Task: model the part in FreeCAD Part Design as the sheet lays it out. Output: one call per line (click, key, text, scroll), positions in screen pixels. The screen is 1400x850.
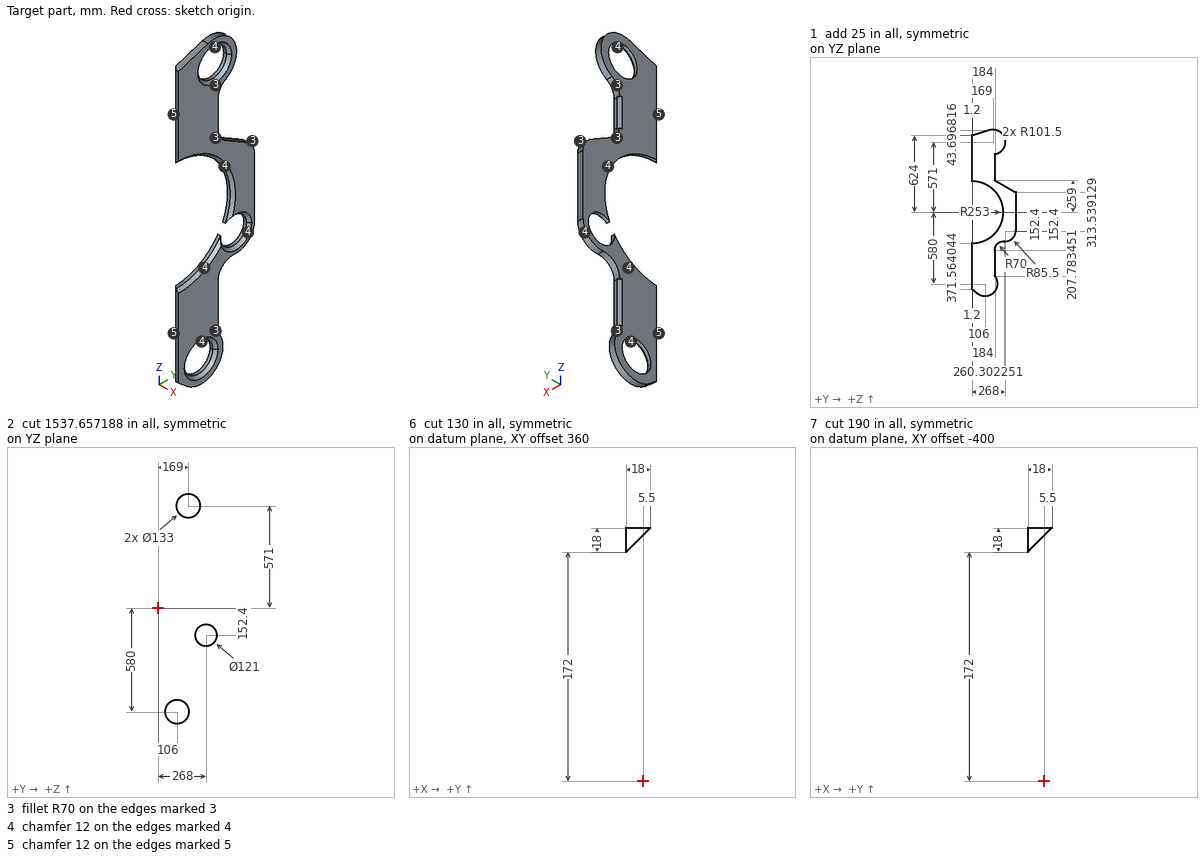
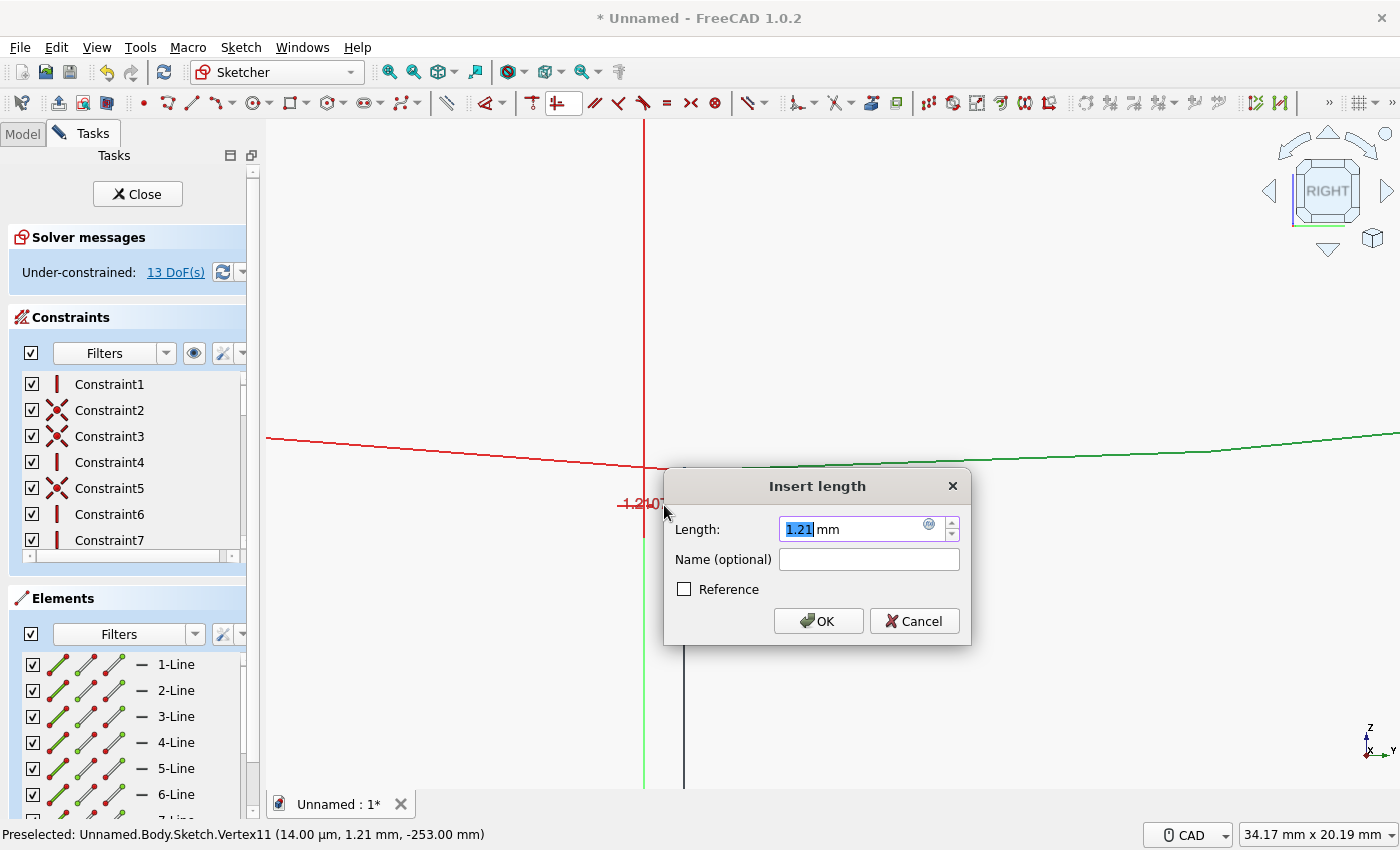
text(1.2)
key(Return)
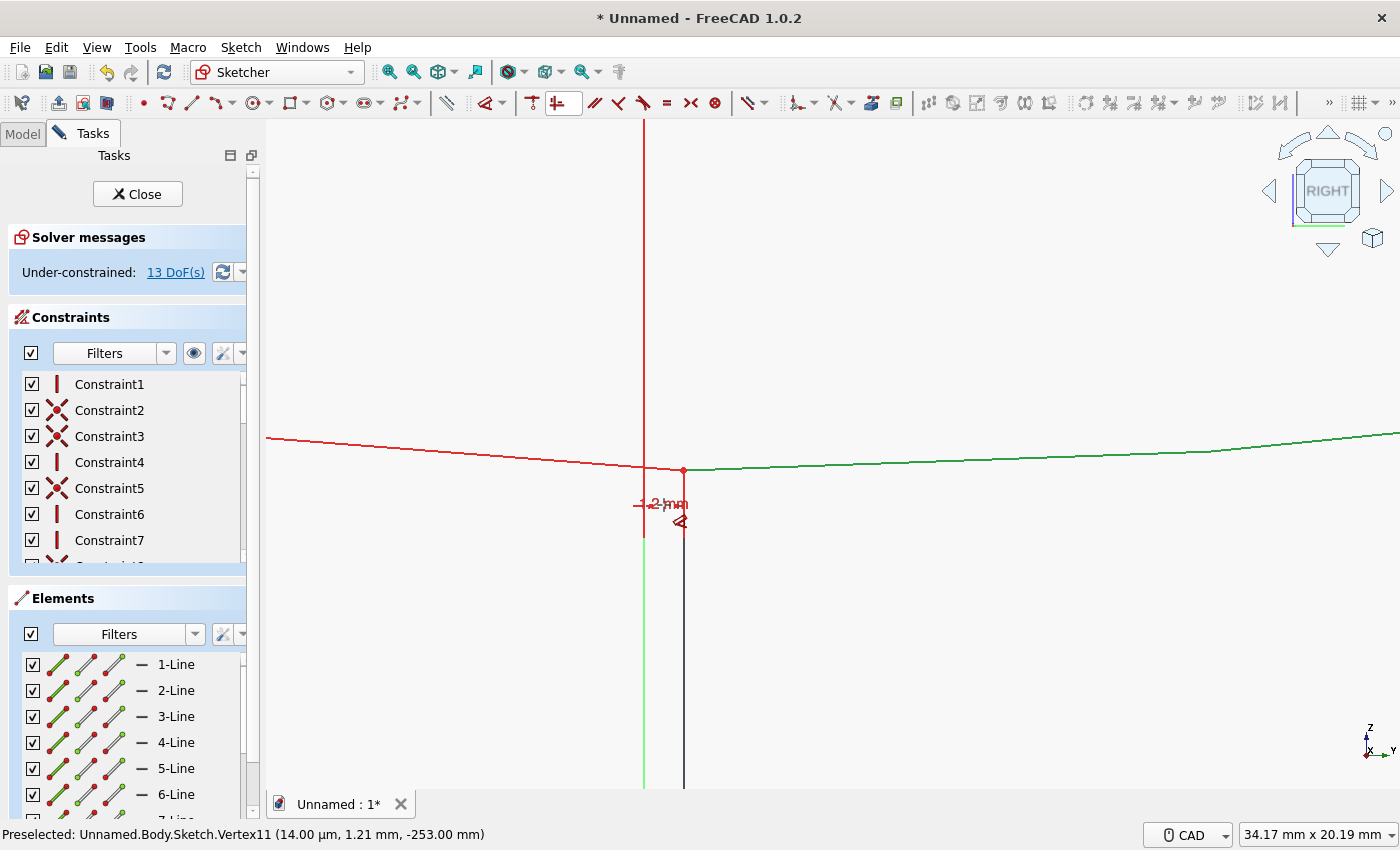
scroll(764, 454, down, 15)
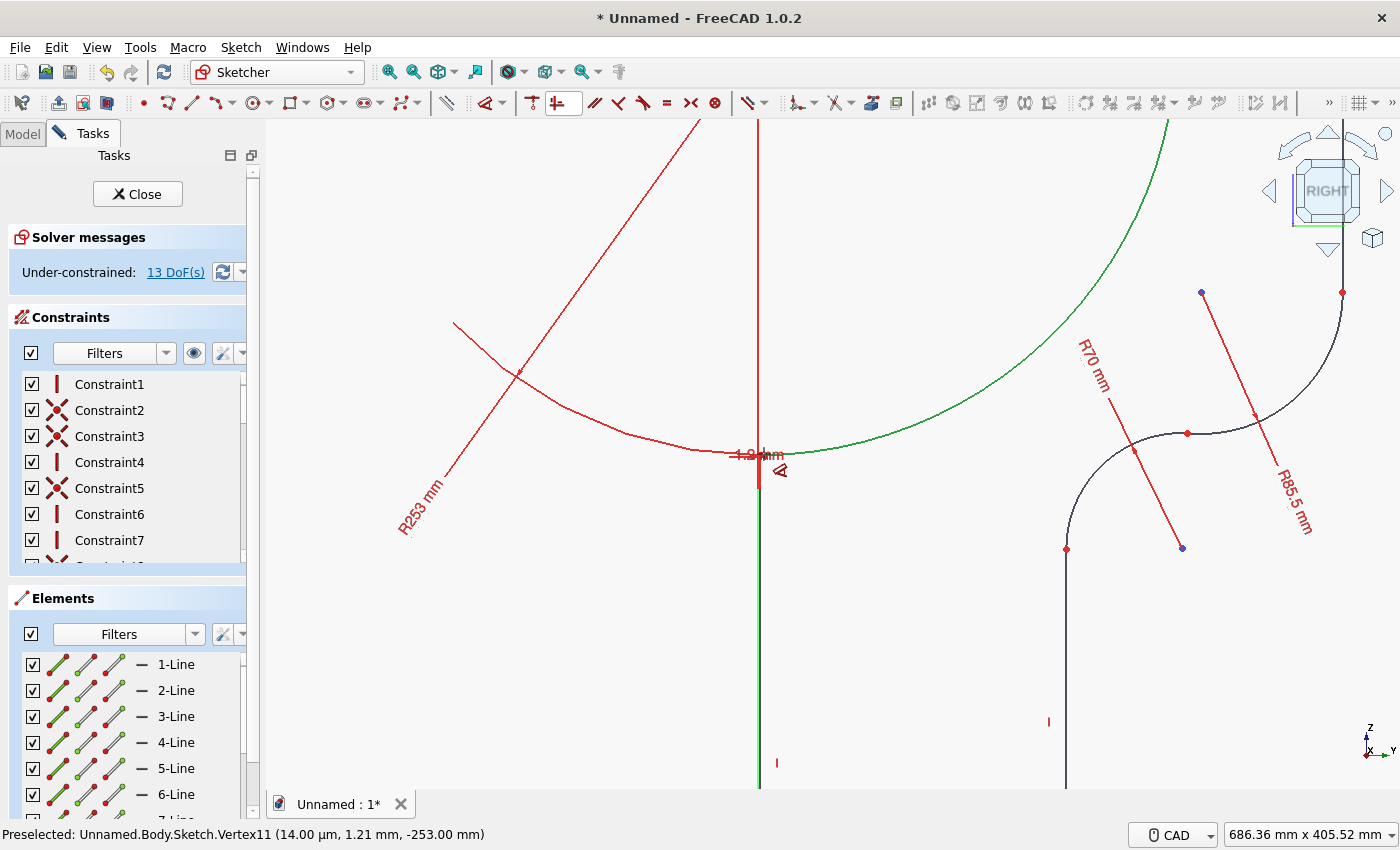
scroll(692, 561, down, 8)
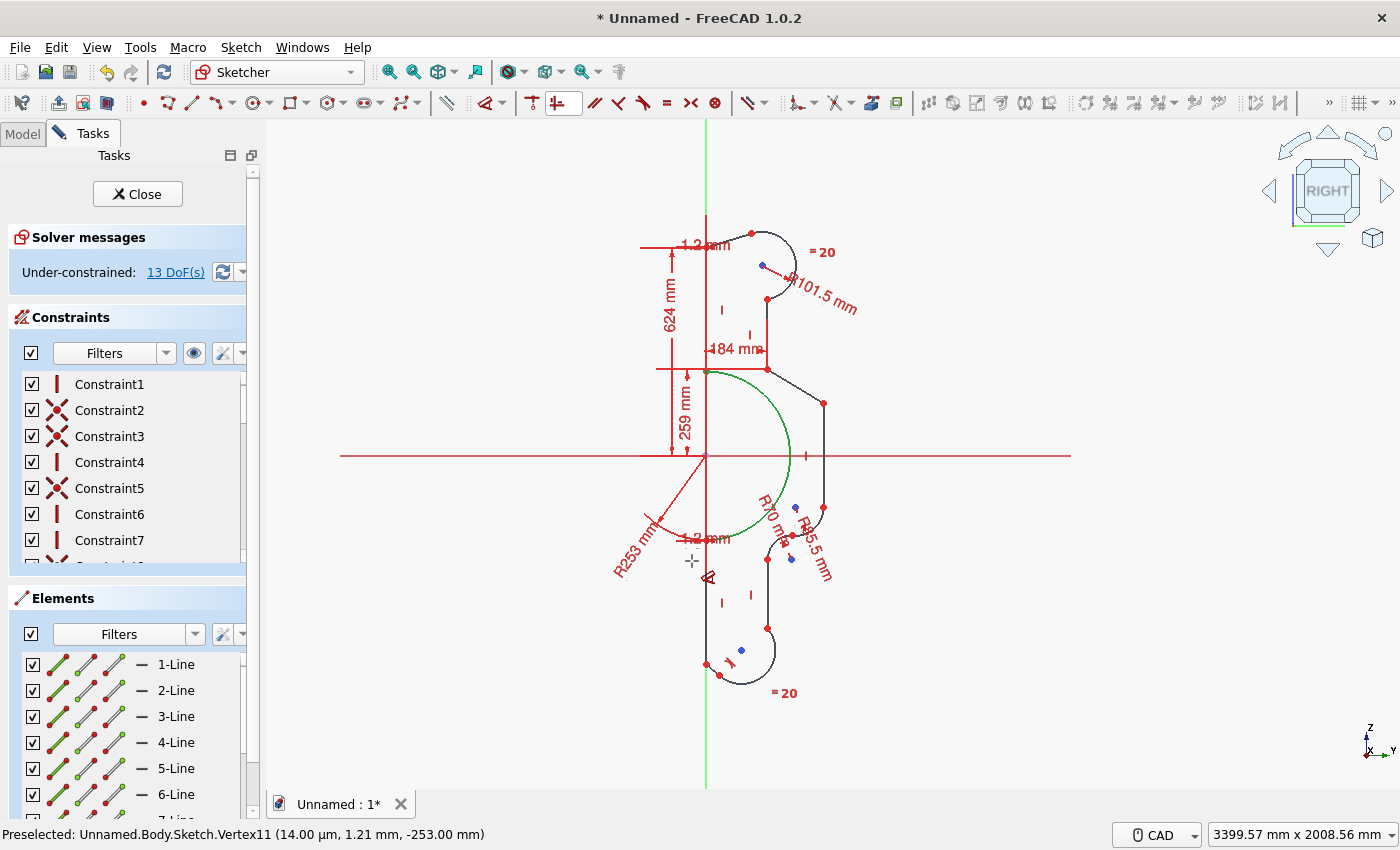
click(768, 629)
click(737, 663)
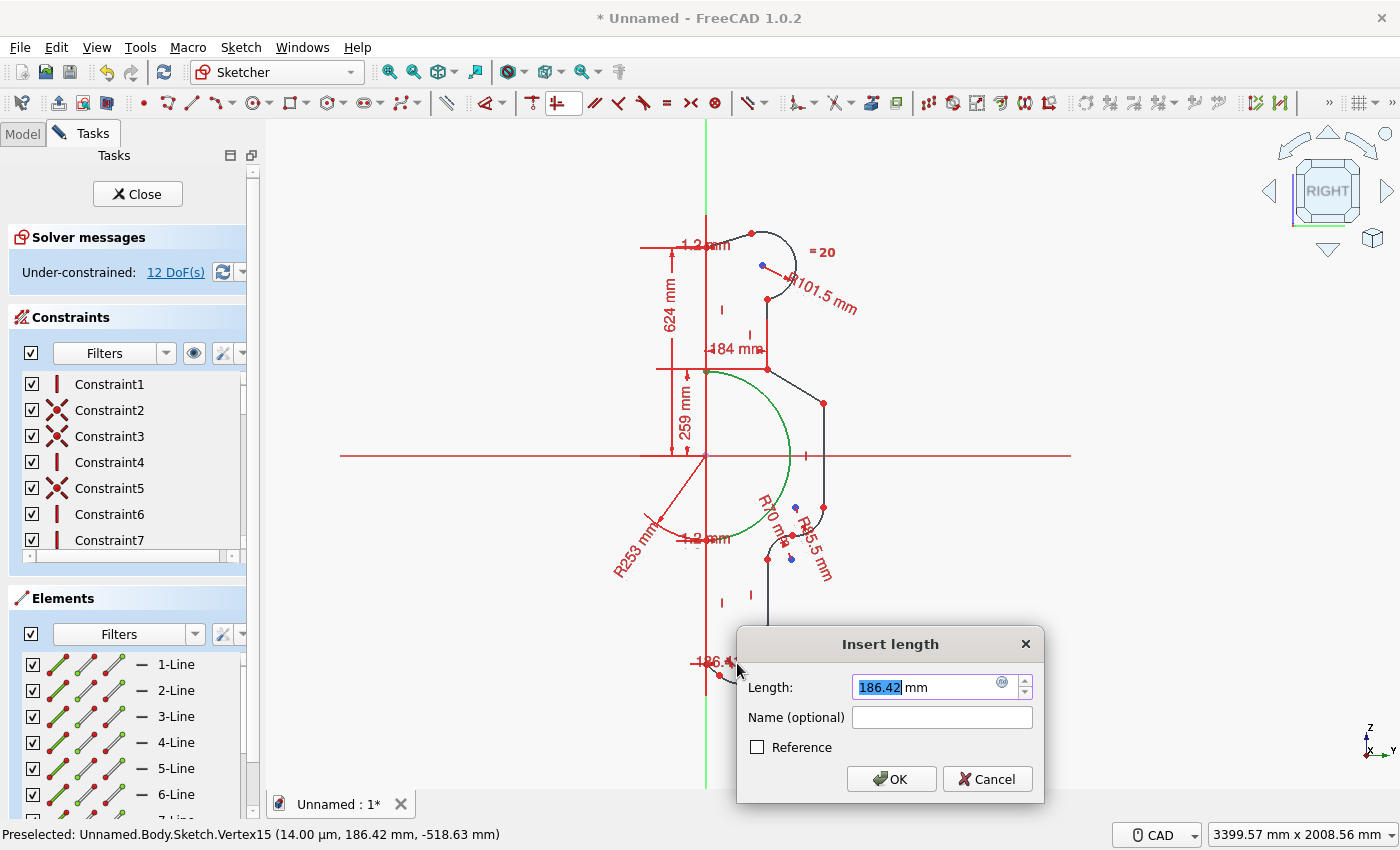
text(184)
key(Return)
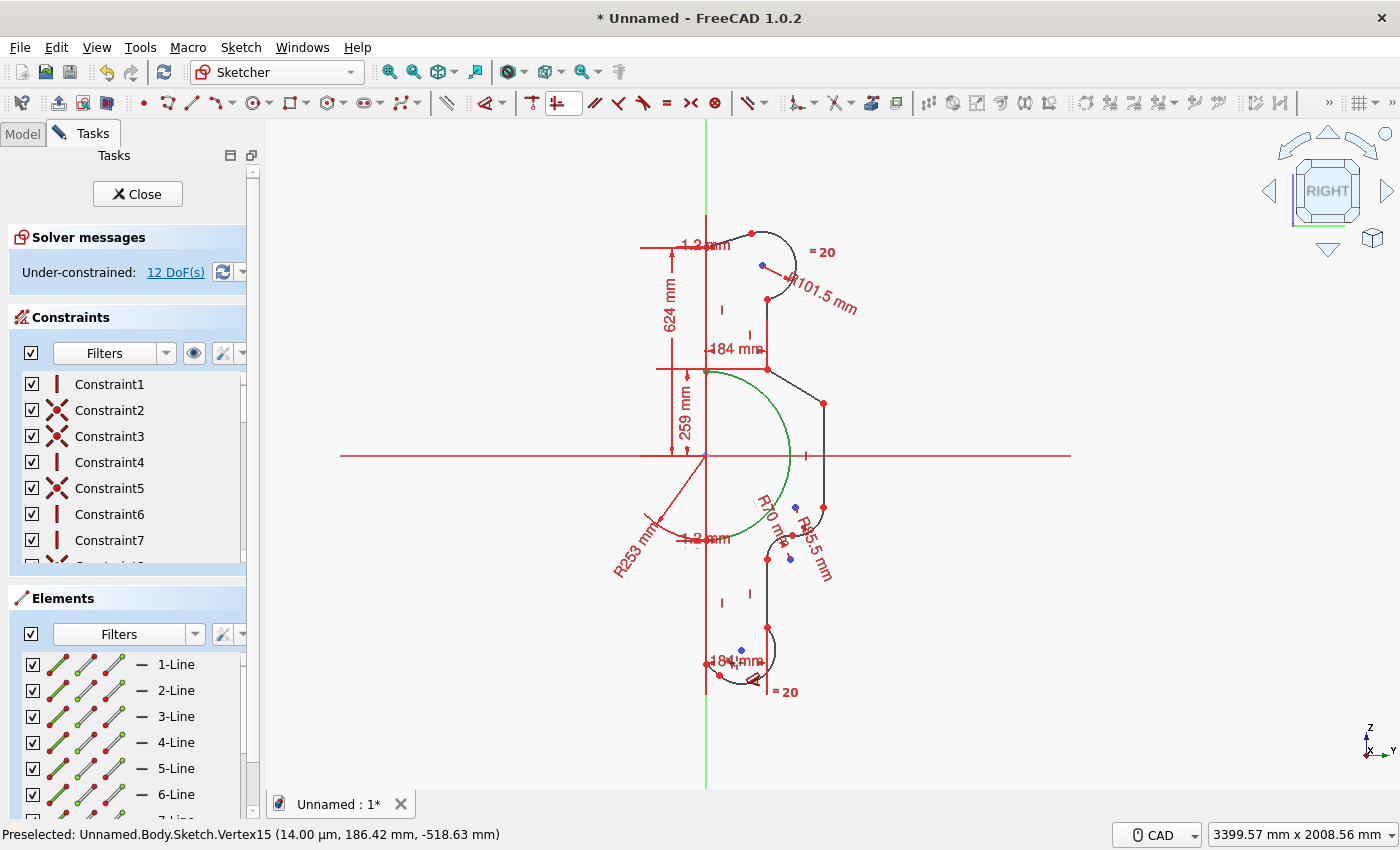
click(762, 266)
click(734, 490)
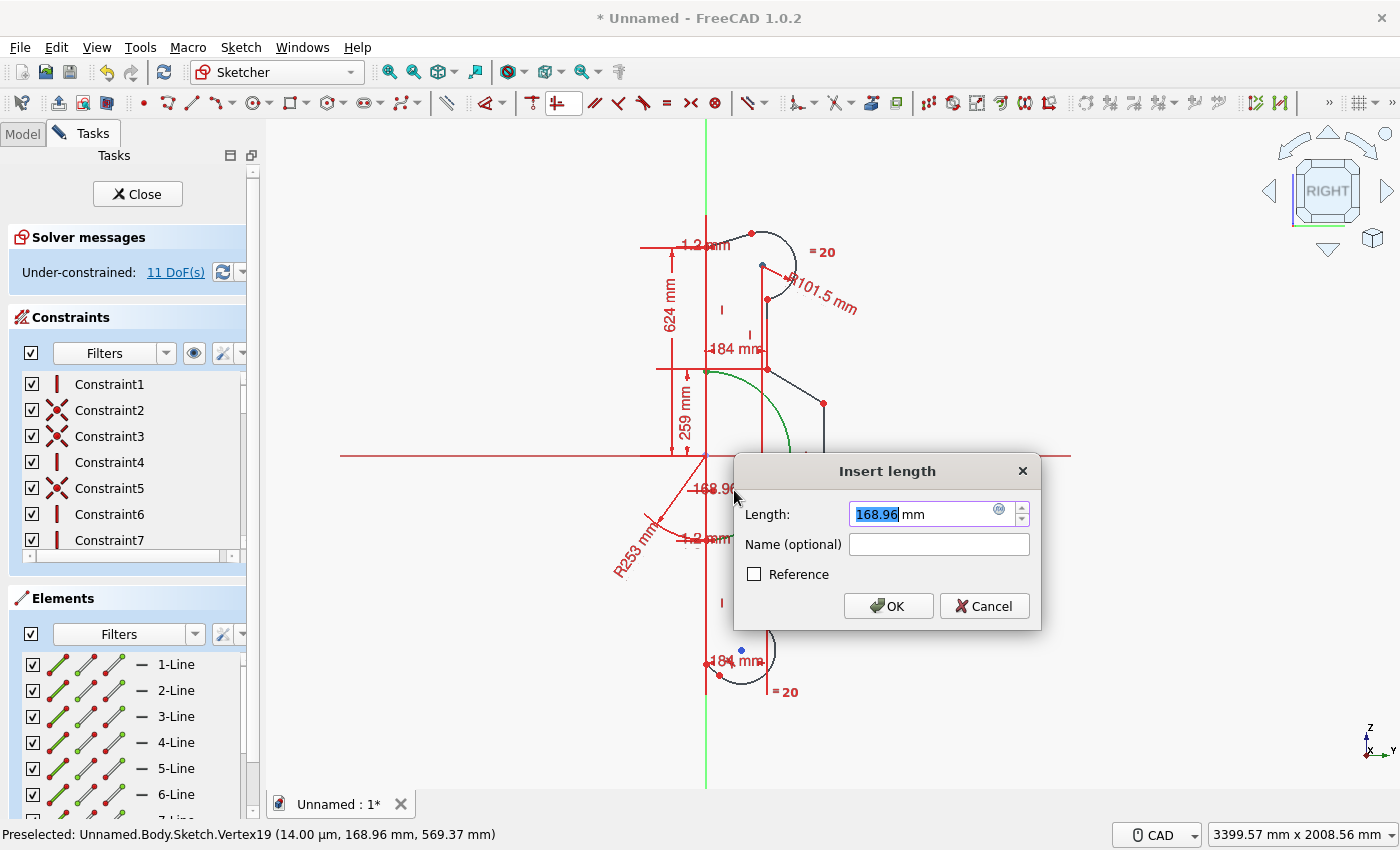
text(169)
key(Return)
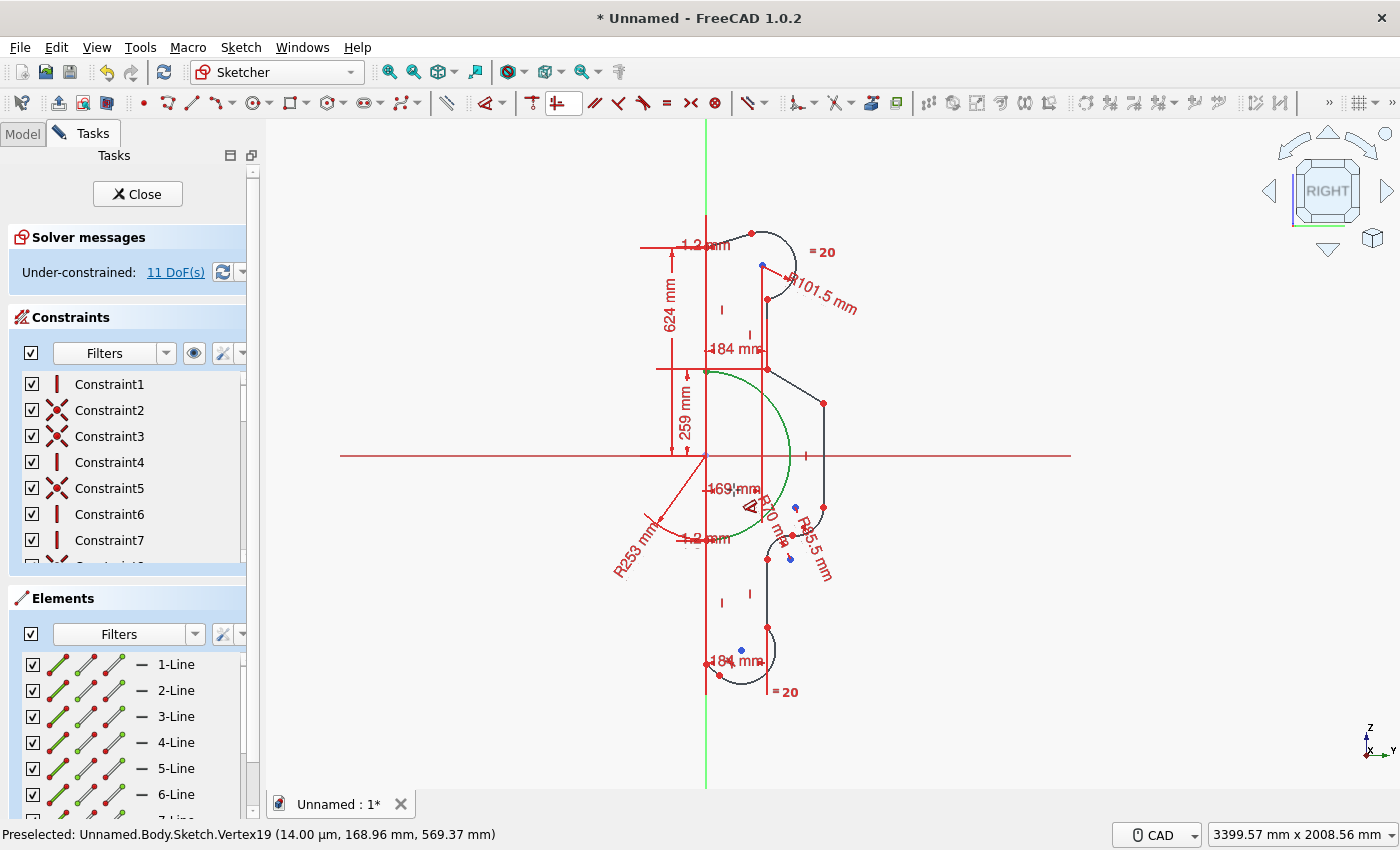
click(762, 266)
click(796, 317)